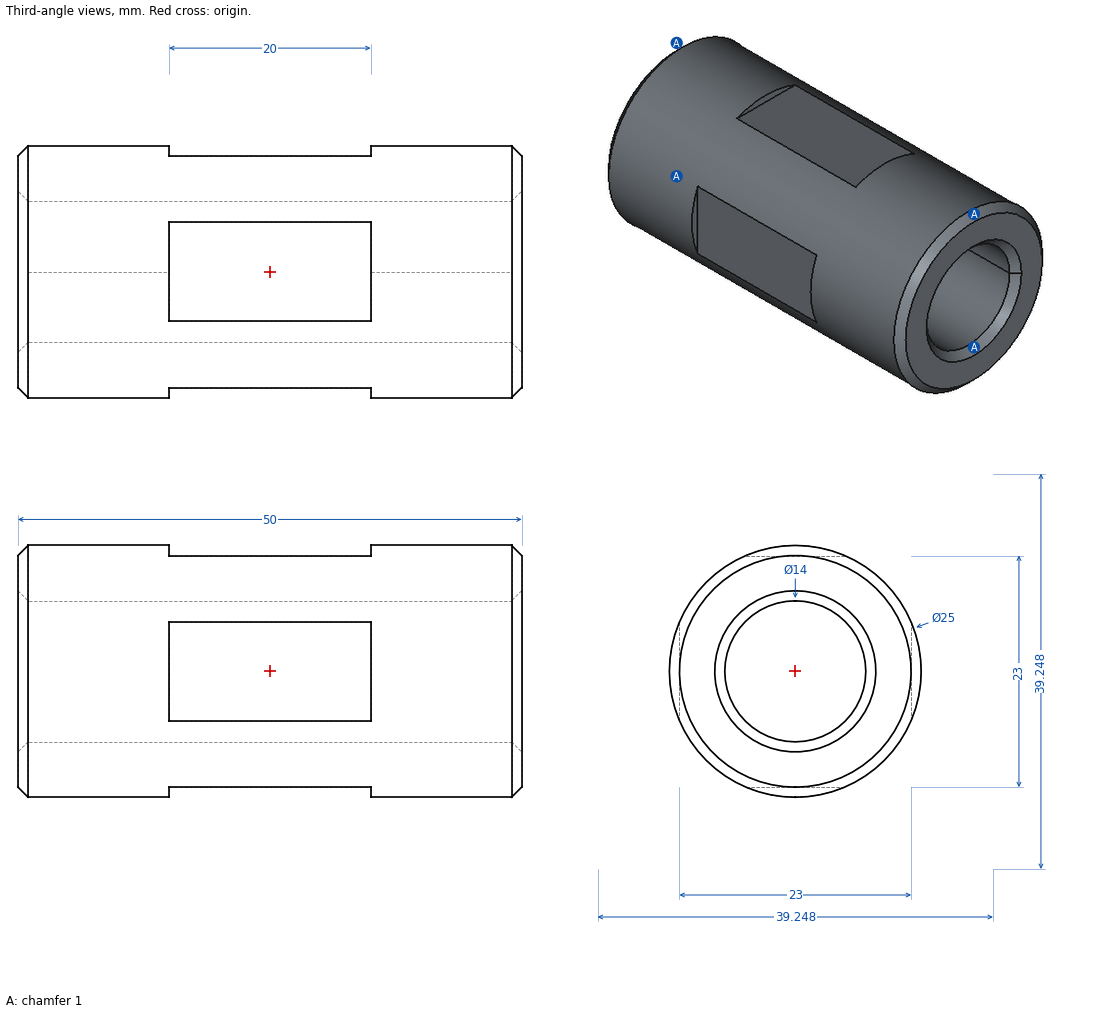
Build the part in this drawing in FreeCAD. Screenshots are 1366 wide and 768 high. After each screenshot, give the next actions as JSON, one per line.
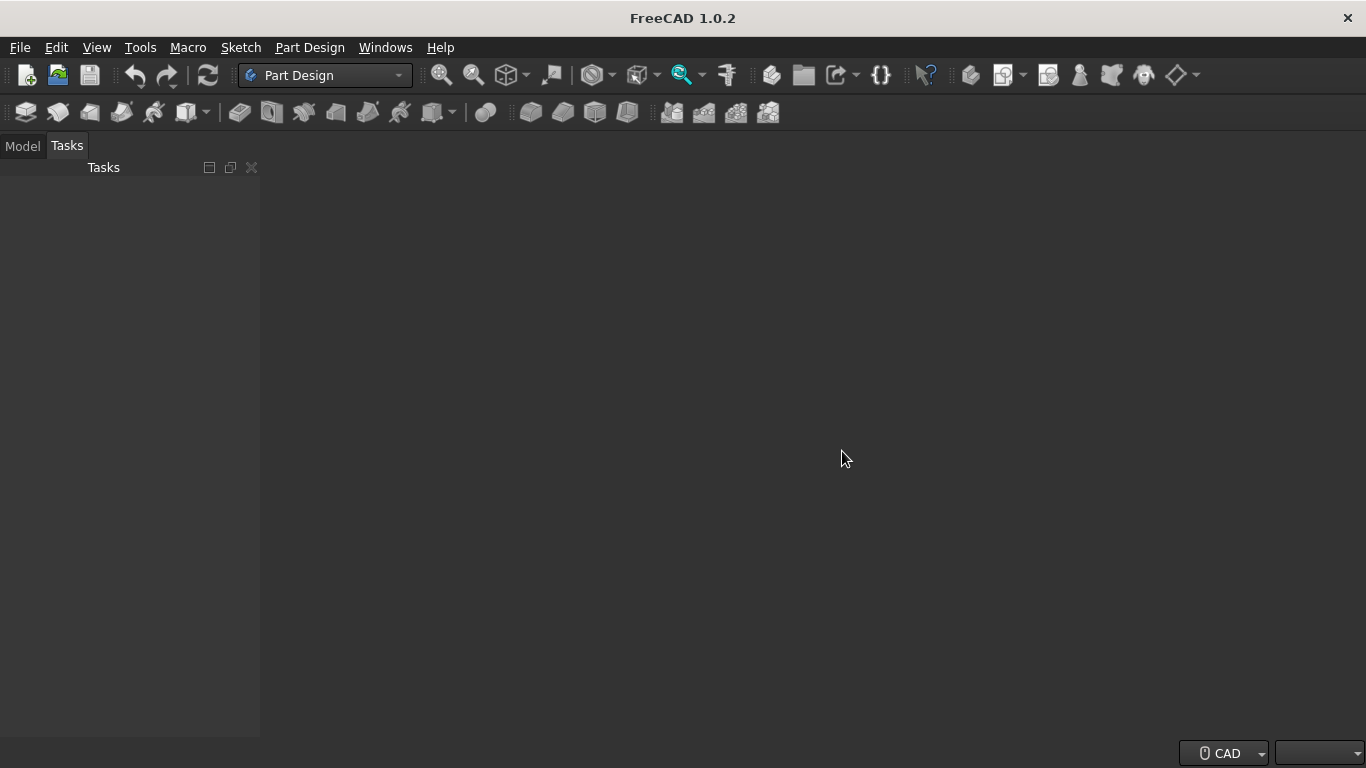
{"action": "key", "text": "ctrl+n"}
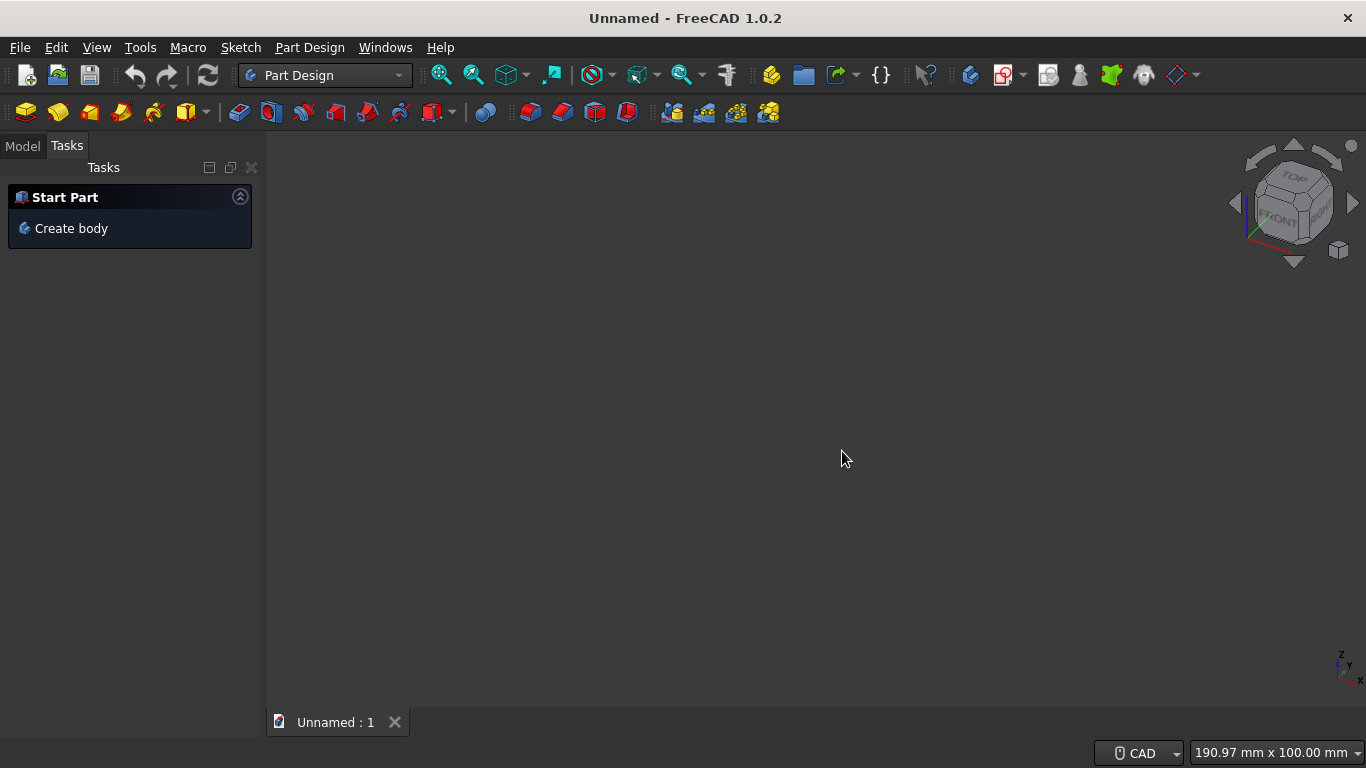
{"action": "left_click", "coordinate": [1004, 76]}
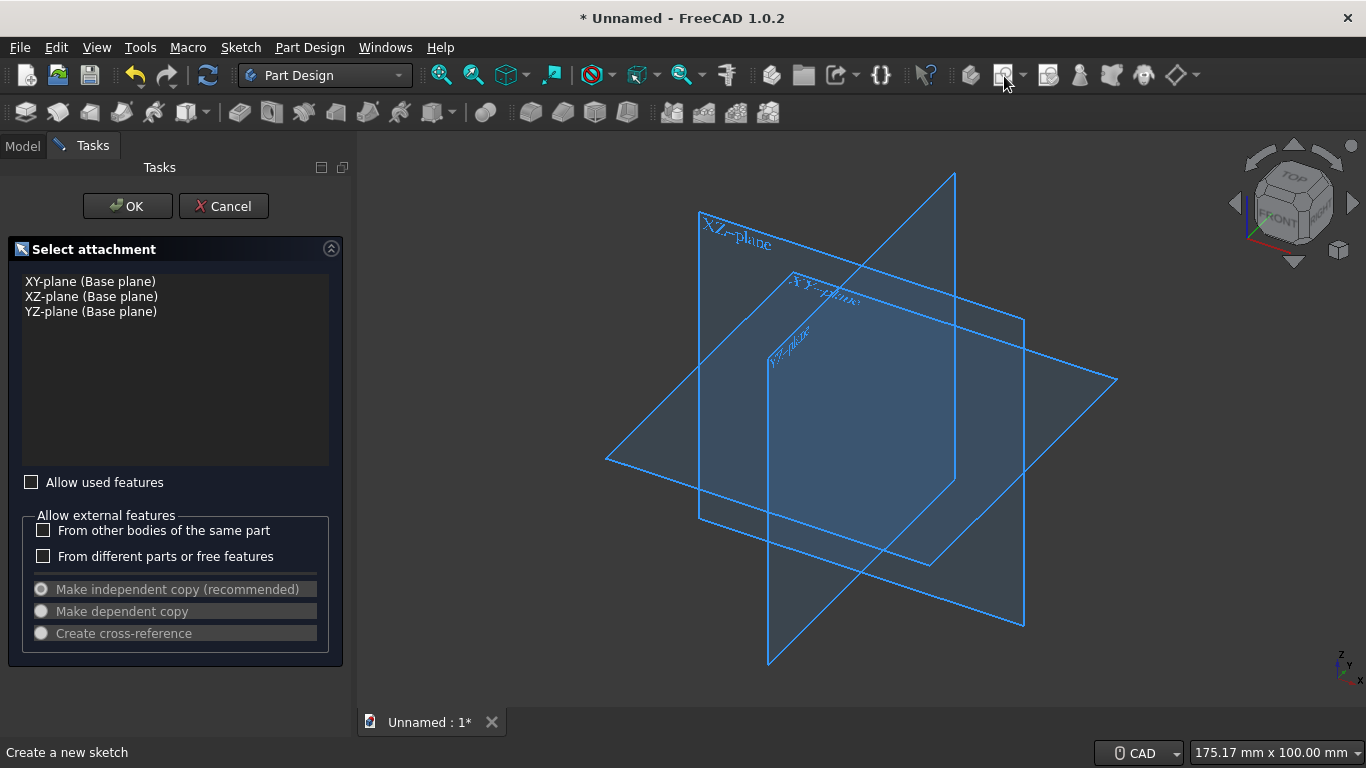
{"action": "left_click", "coordinate": [82, 312]}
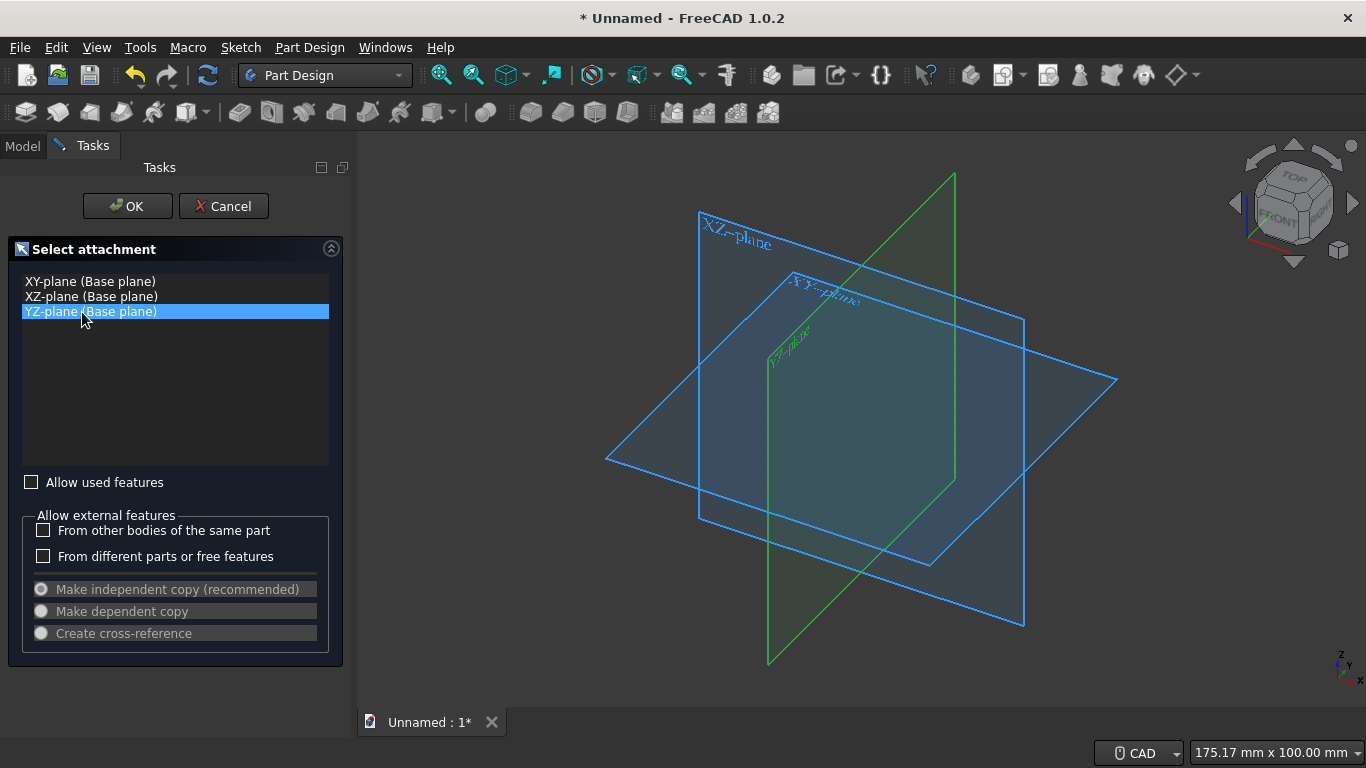
{"action": "left_click", "coordinate": [128, 206]}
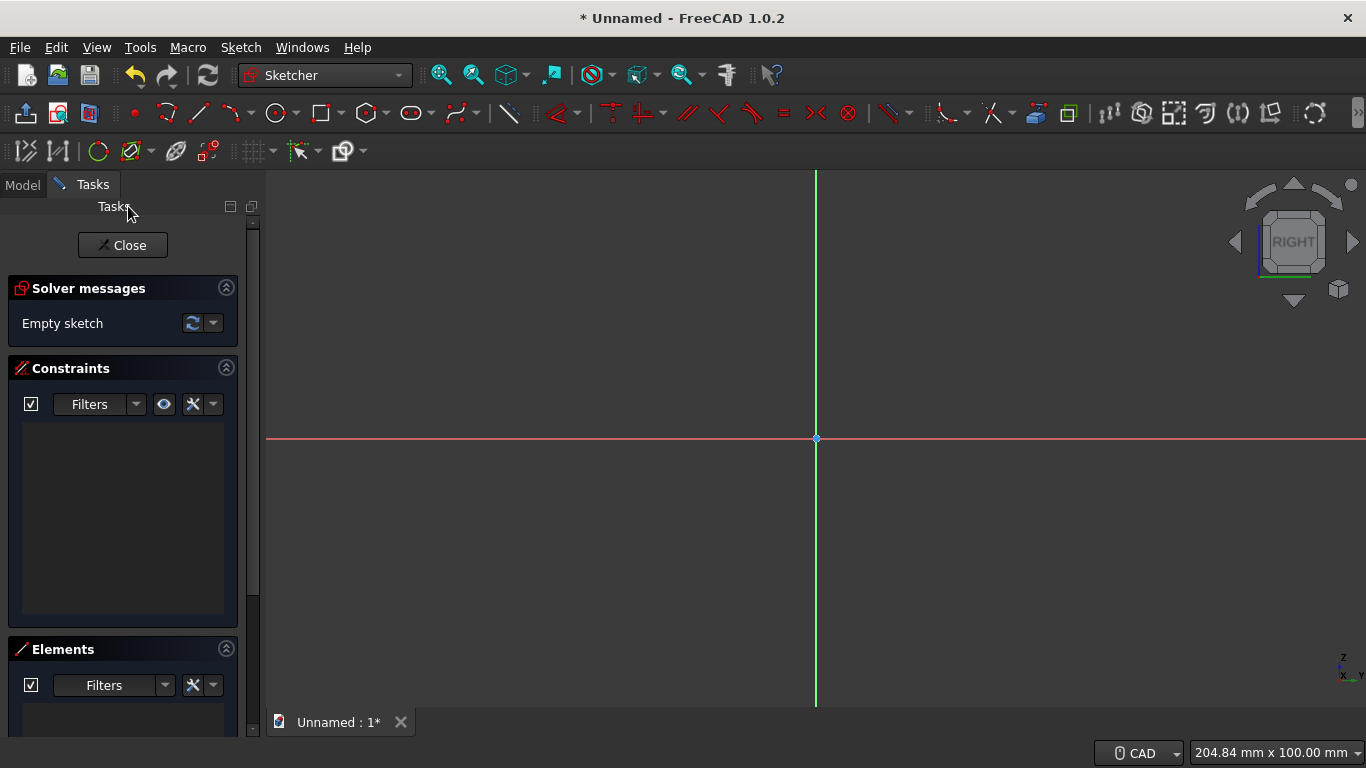
{"action": "scroll", "coordinate": [856, 439], "scroll_direction": "up", "scroll_amount": 5}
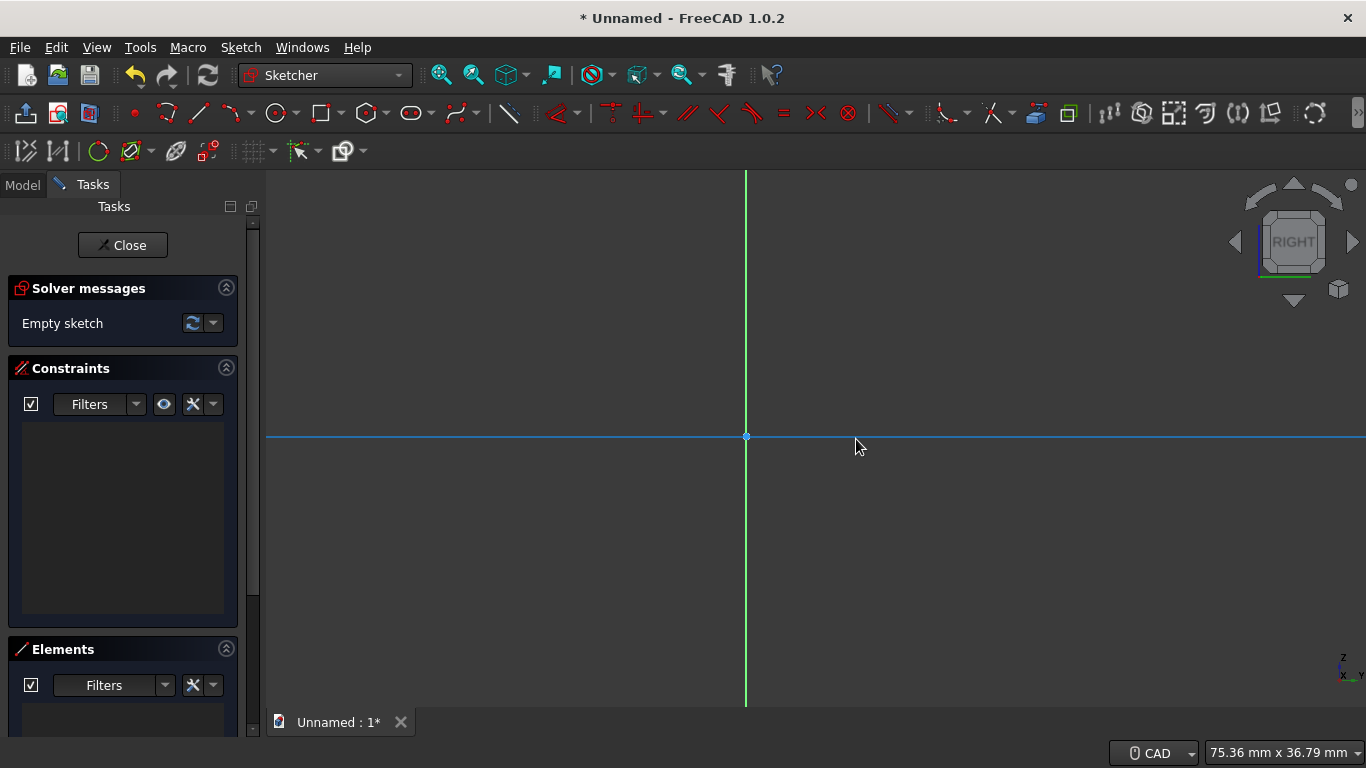
{"action": "left_click", "coordinate": [276, 114]}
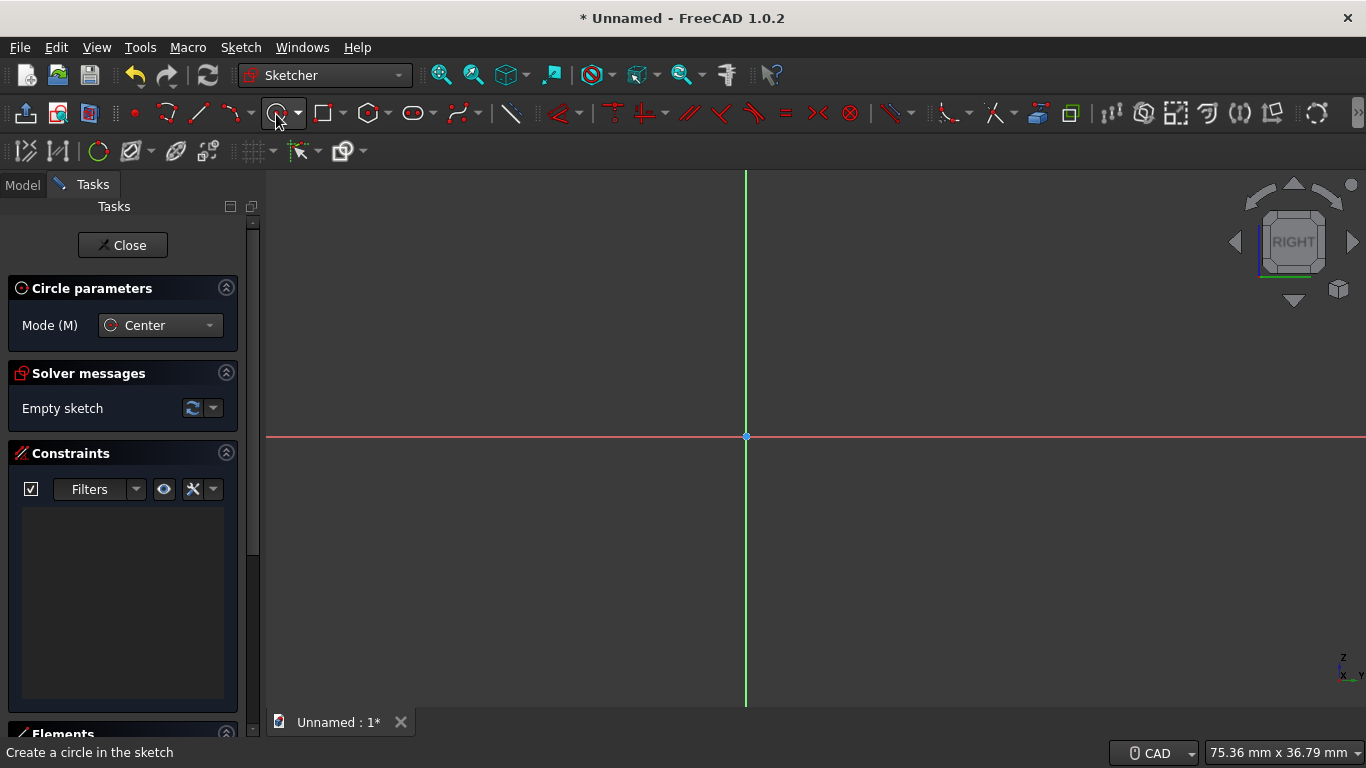
{"action": "left_click", "coordinate": [746, 437]}
{"action": "mouse_move", "coordinate": [875, 308]}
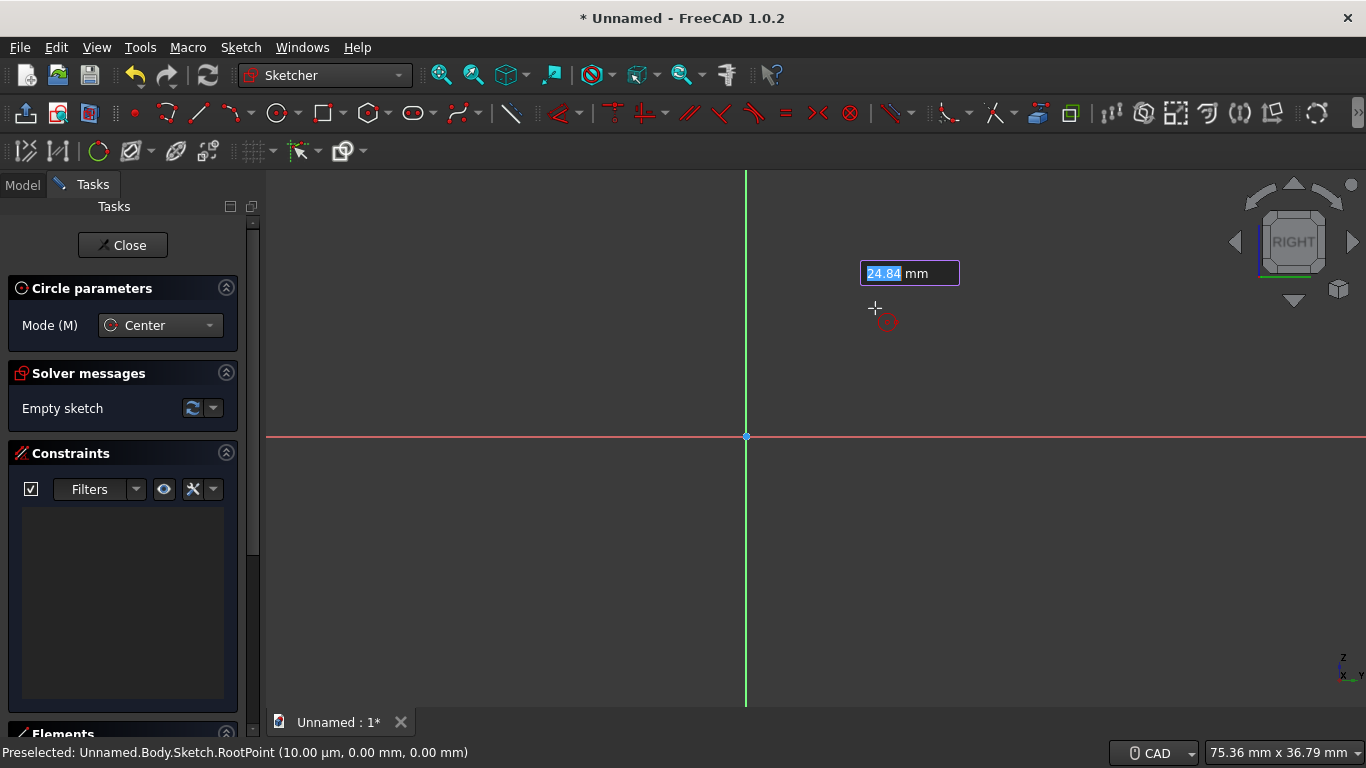
{"action": "type", "text": "25"}
{"action": "key", "text": "Return"}
{"action": "key", "text": "Escape"}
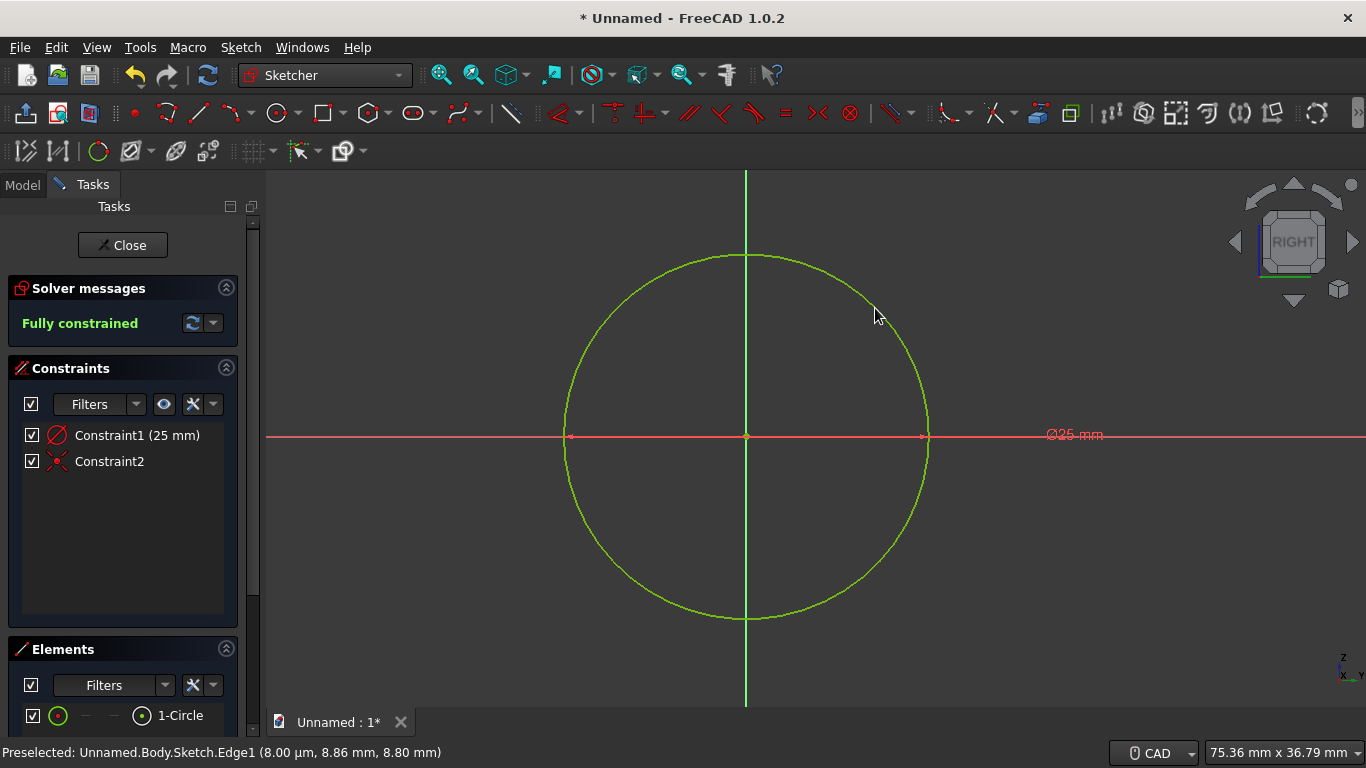
{"action": "left_click", "coordinate": [123, 245]}